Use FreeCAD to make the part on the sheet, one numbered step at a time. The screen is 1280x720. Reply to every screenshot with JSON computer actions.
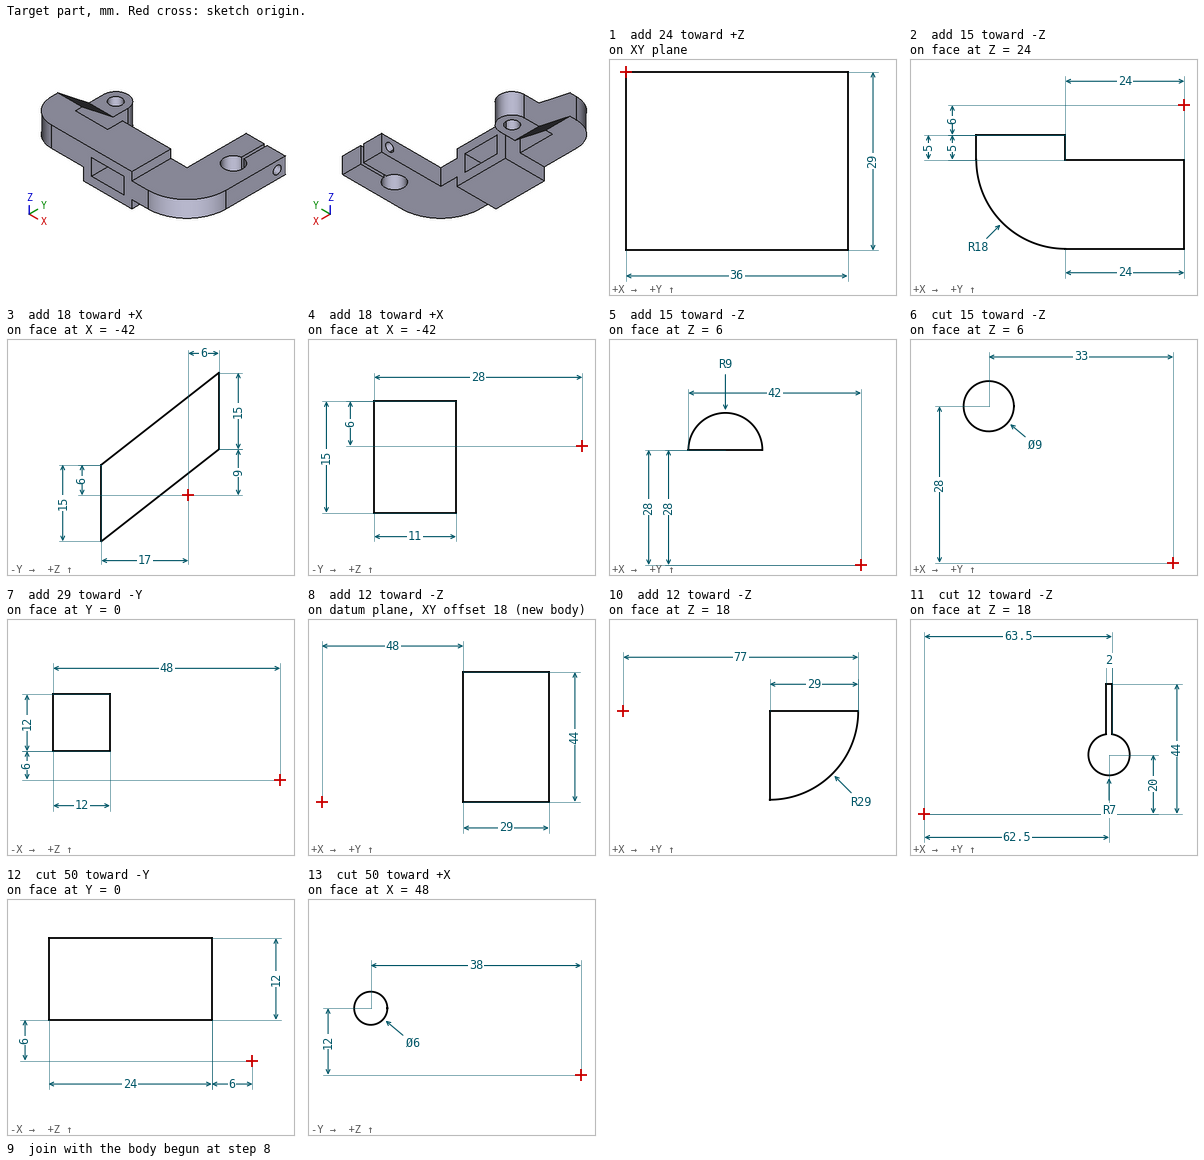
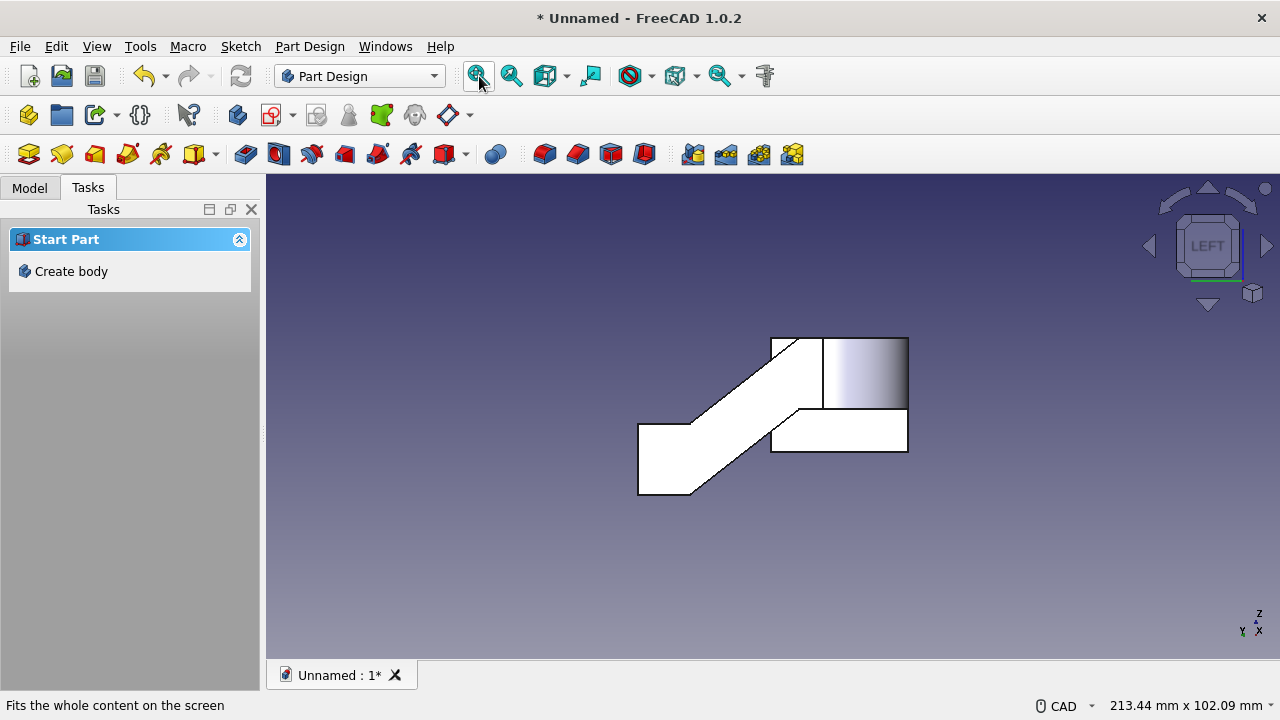
{"action": "key", "text": "0"}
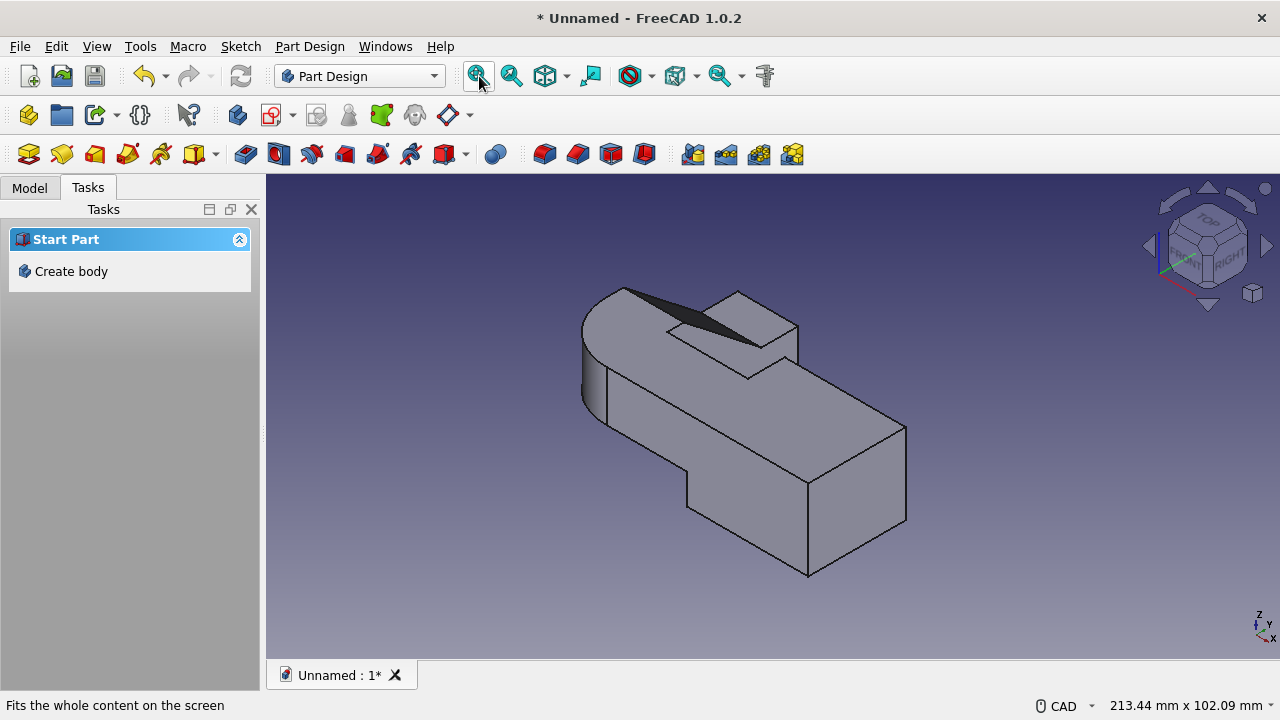
{"action": "left_click", "coordinate": [758, 324]}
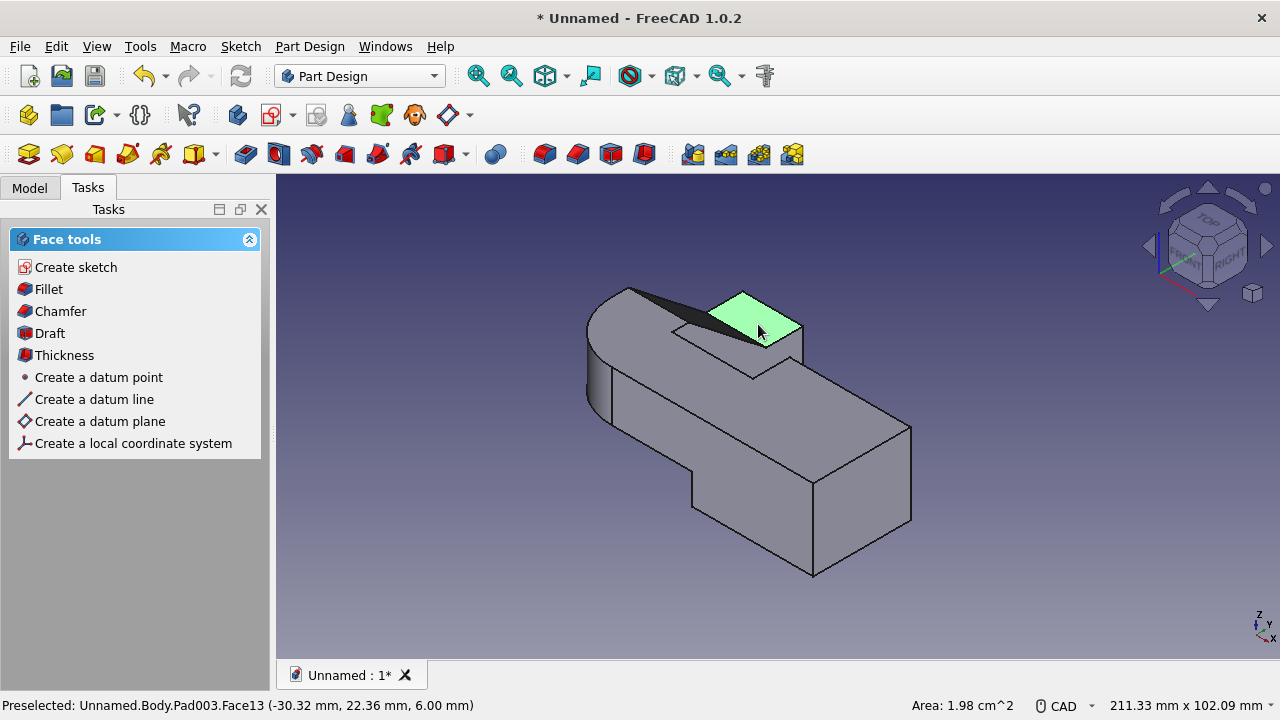
{"action": "left_click", "coordinate": [270, 116]}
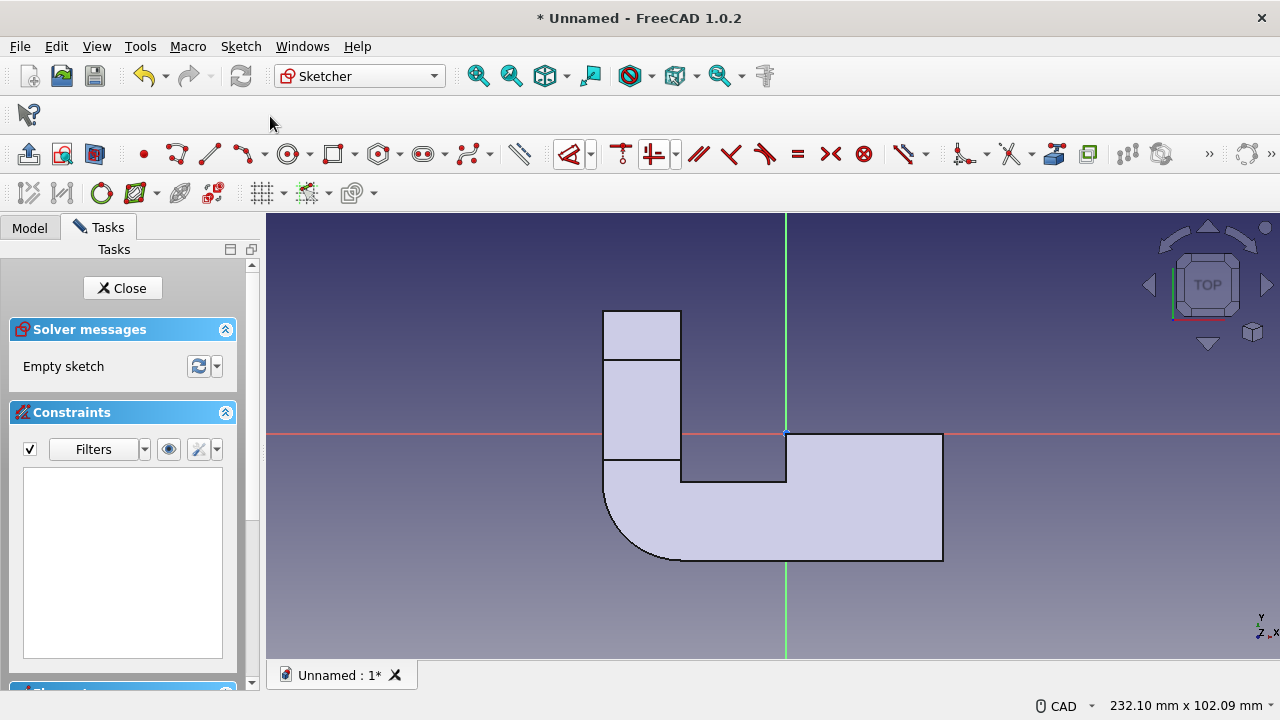
{"action": "left_click", "coordinate": [95, 154]}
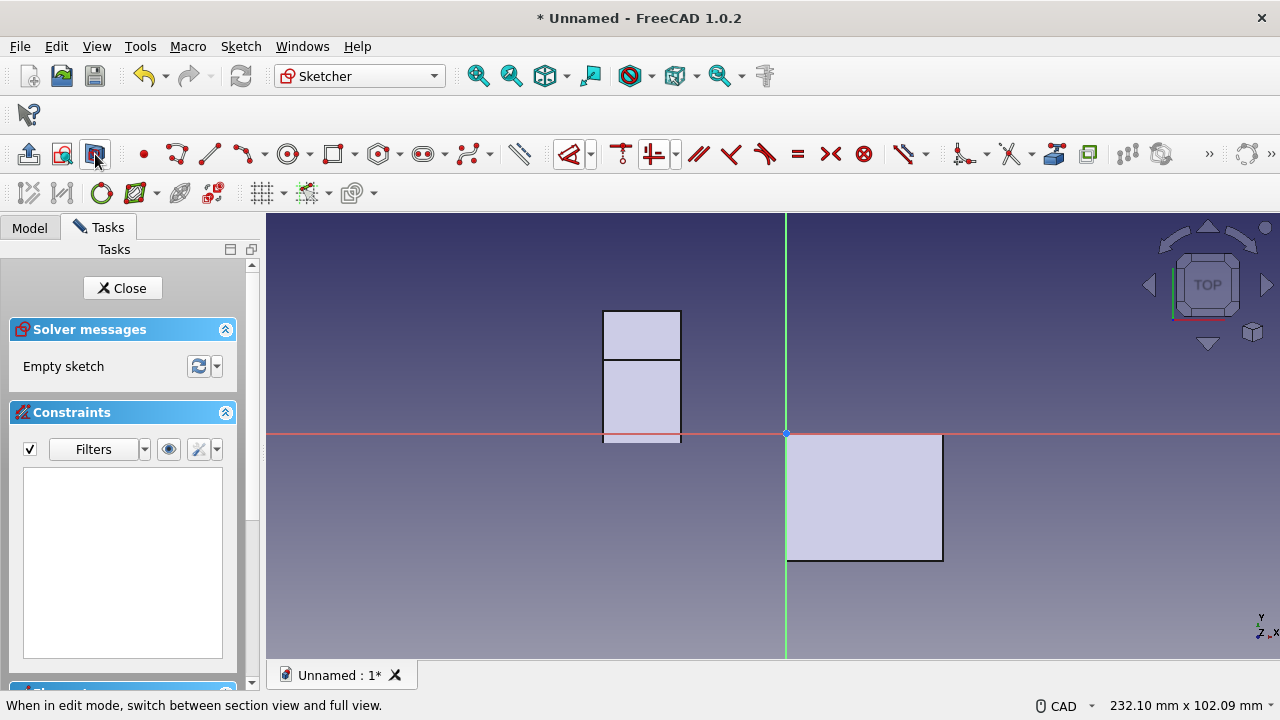
{"action": "scroll", "coordinate": [682, 252], "scroll_direction": "up", "scroll_amount": 3}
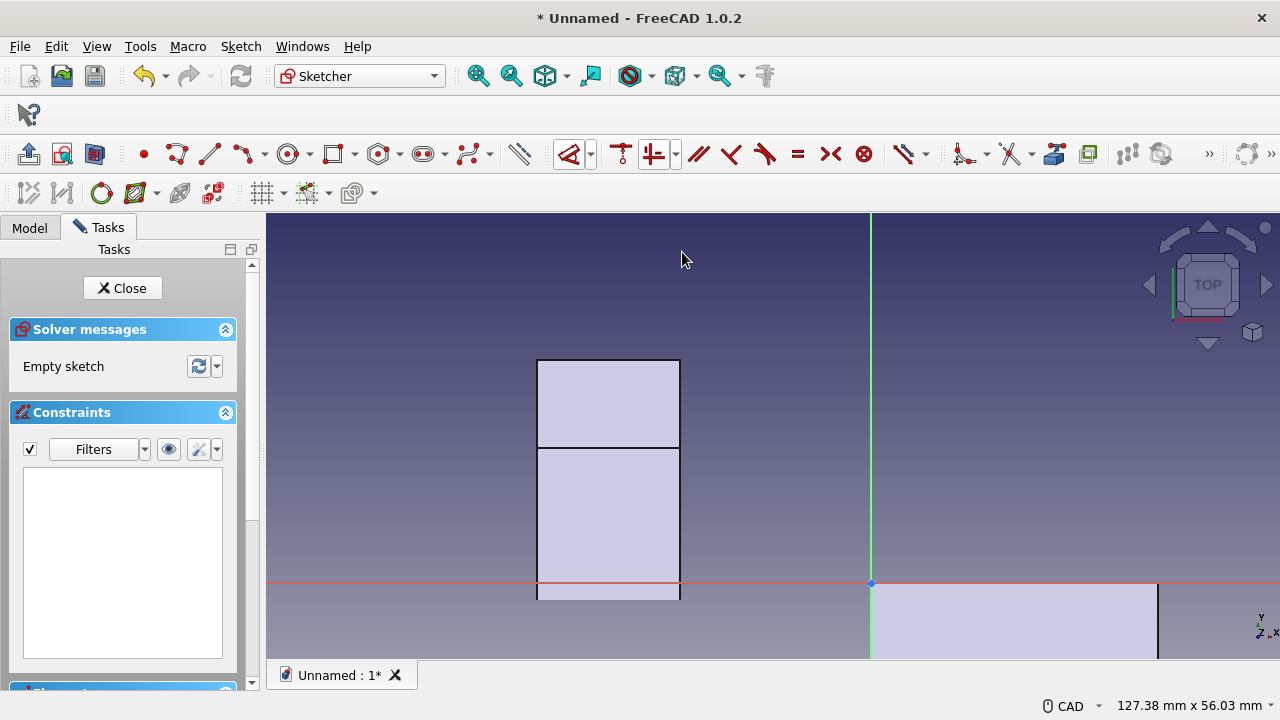
{"action": "left_click", "coordinate": [210, 154]}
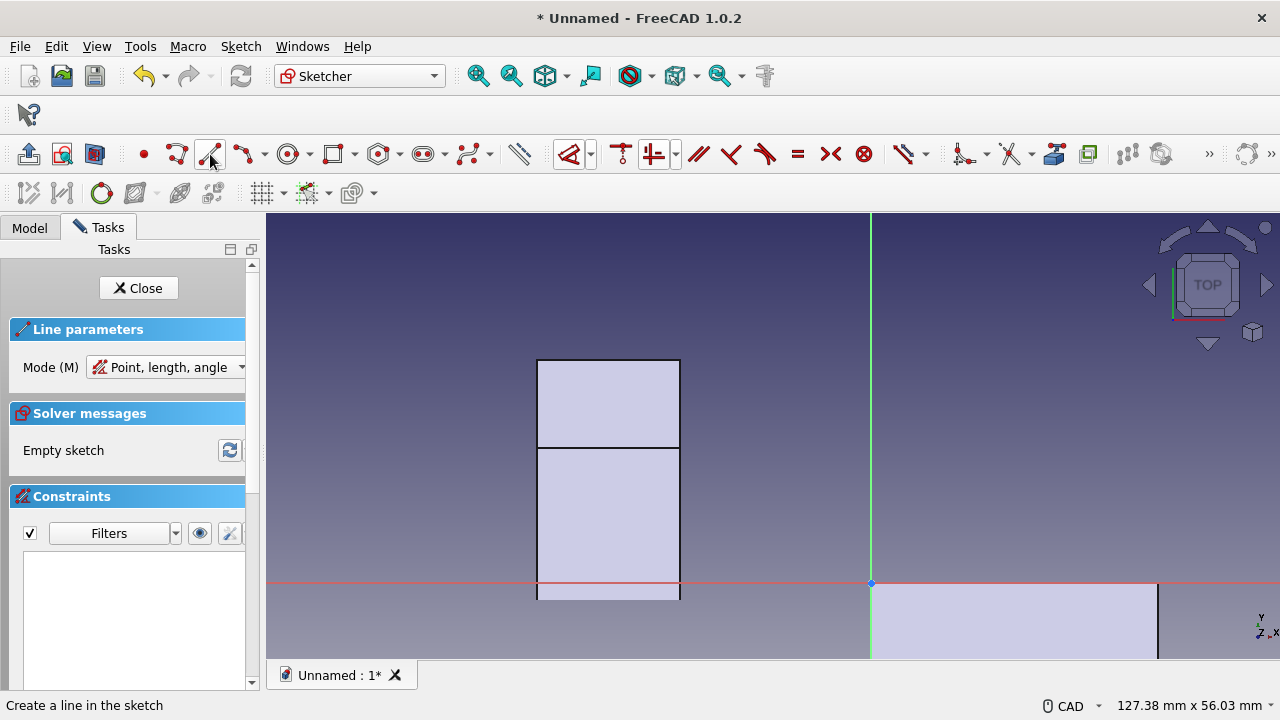
{"action": "left_click", "coordinate": [537, 360]}
{"action": "left_click", "coordinate": [680, 360]}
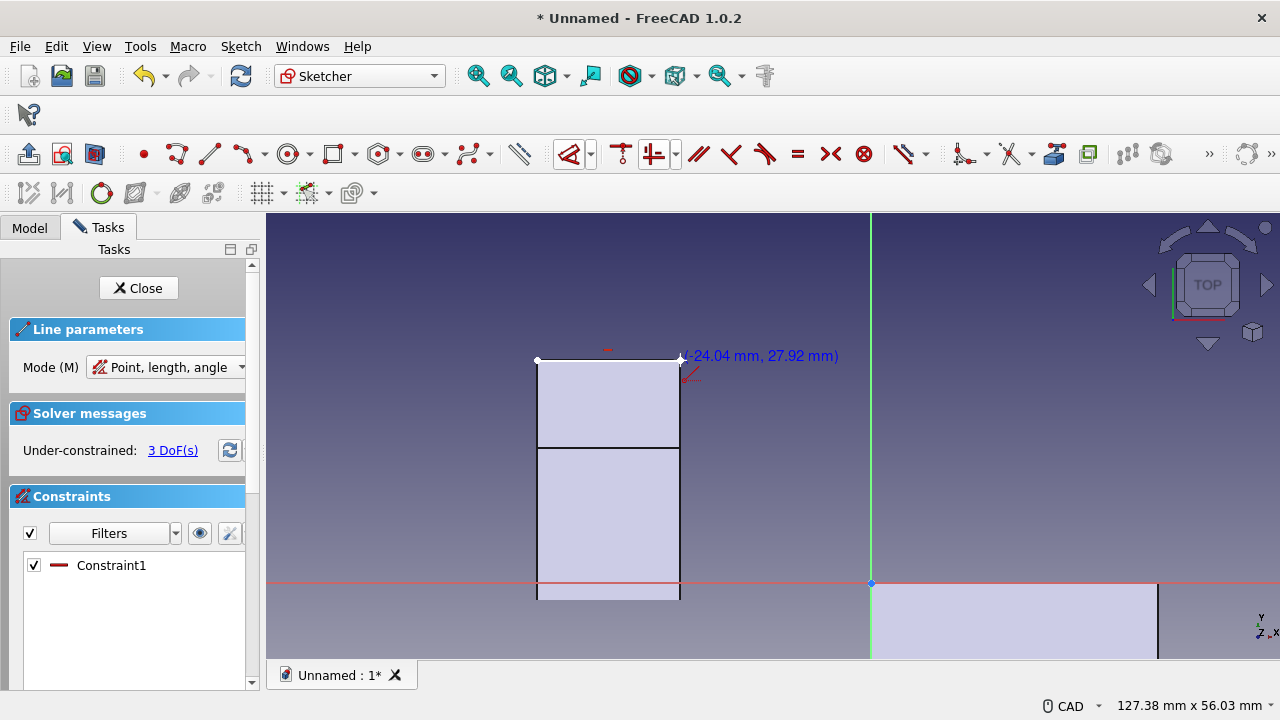
{"action": "key", "text": "g 3 a"}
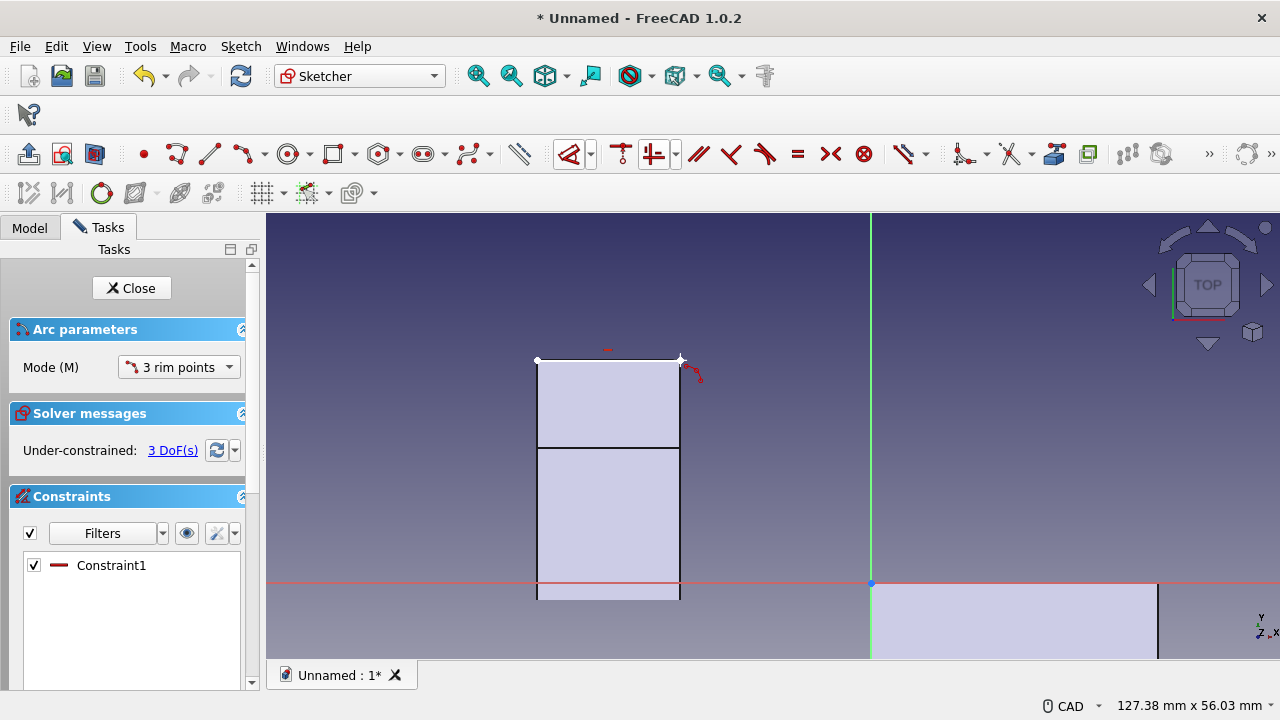
{"action": "left_click", "coordinate": [680, 361]}
{"action": "left_click", "coordinate": [537, 361]}
{"action": "left_click", "coordinate": [609, 289]}
{"action": "key", "text": "Escape"}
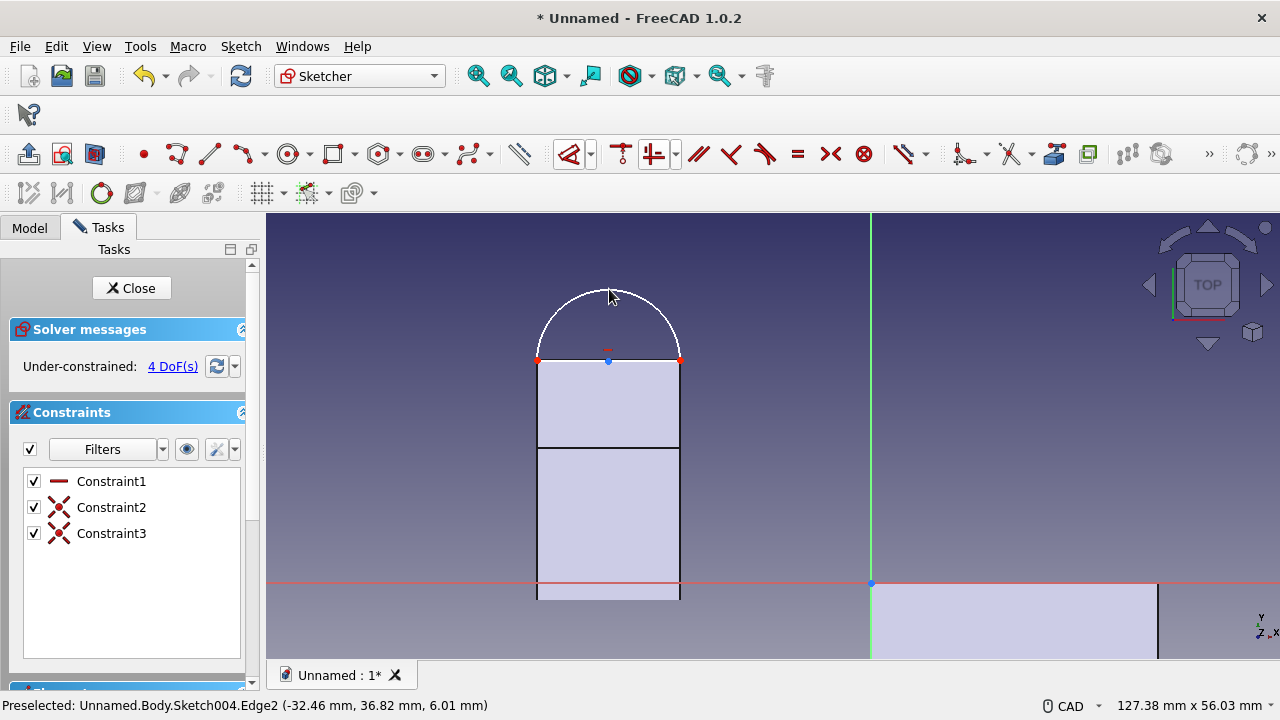
{"action": "left_click", "coordinate": [650, 304]}